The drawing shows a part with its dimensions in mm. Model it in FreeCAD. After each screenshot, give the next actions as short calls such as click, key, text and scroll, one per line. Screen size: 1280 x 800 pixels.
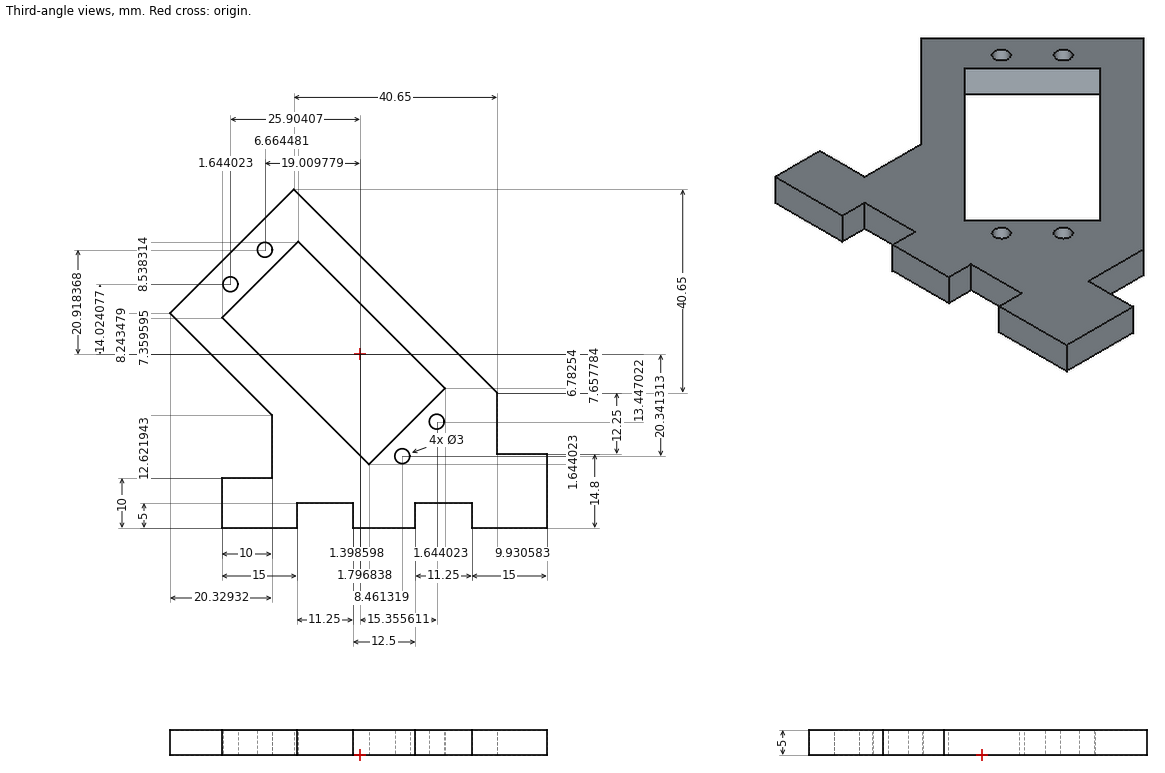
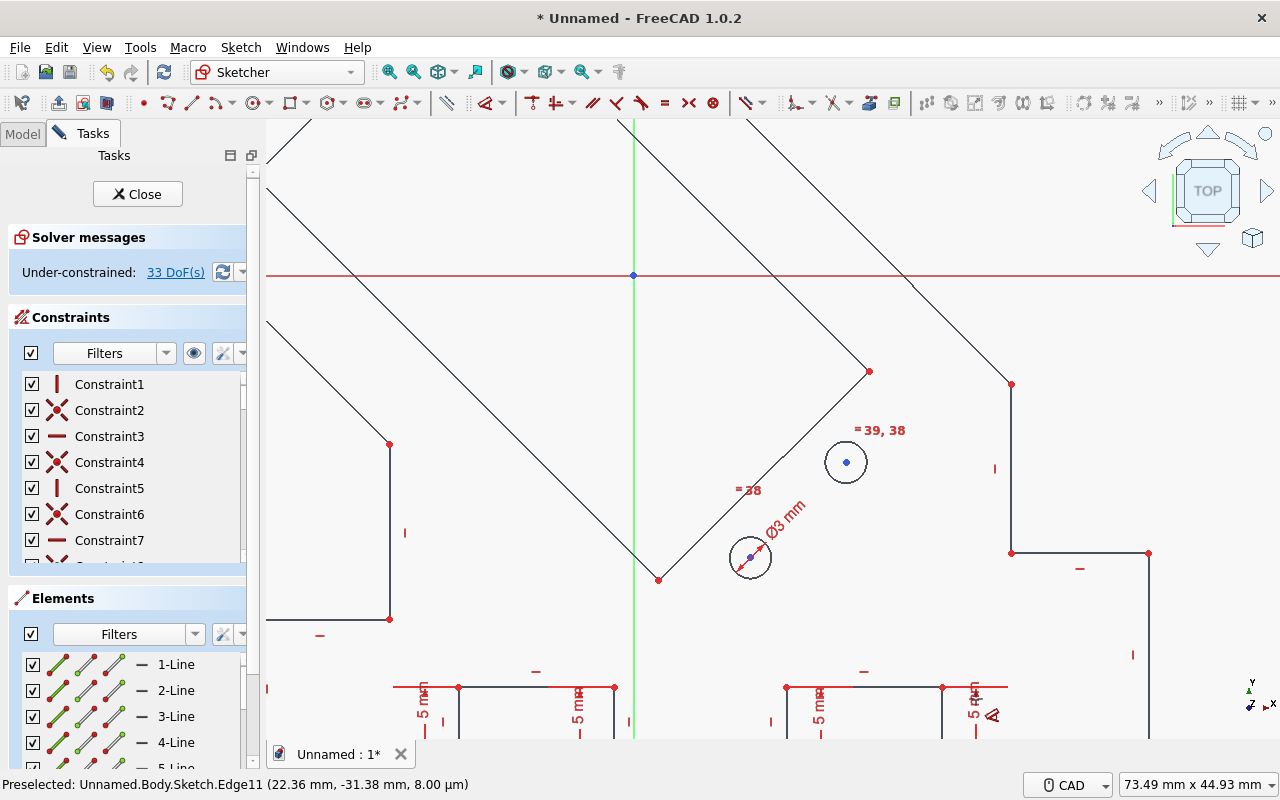
click(348, 620)
click(342, 654)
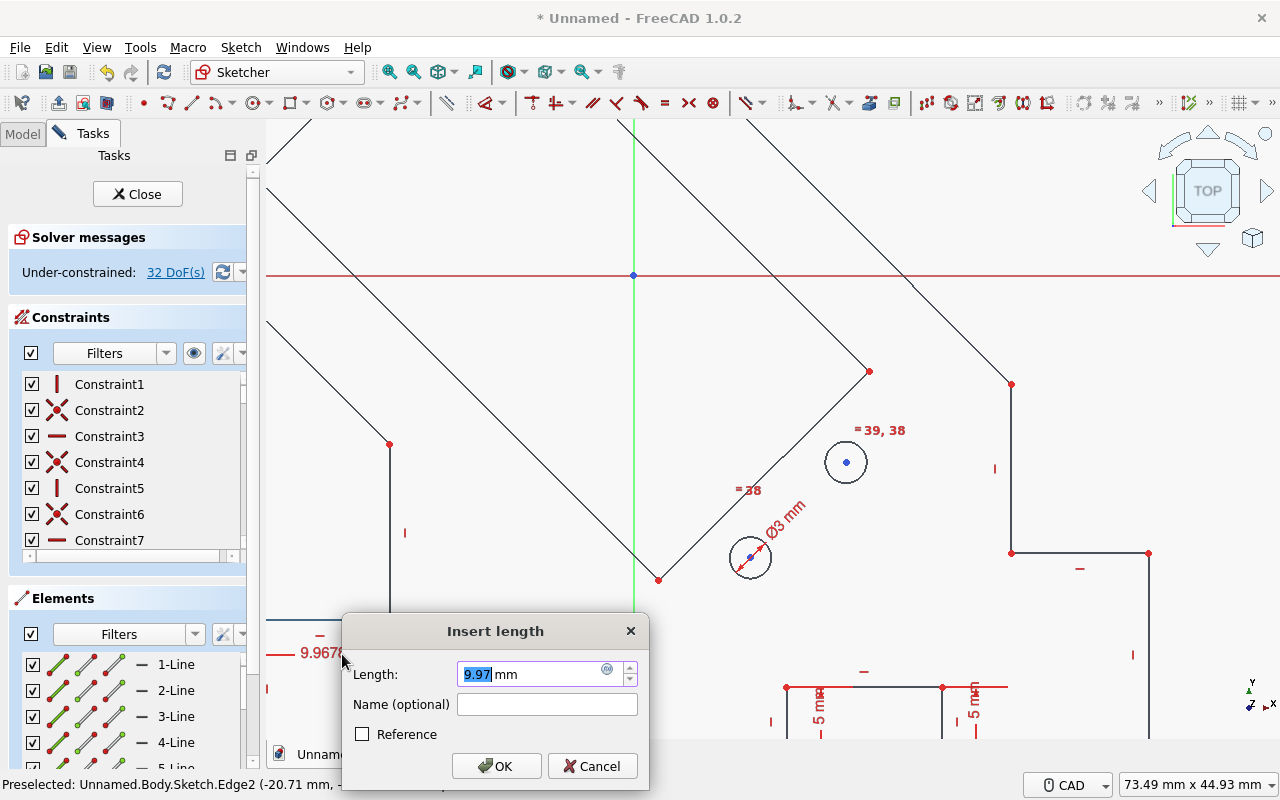
text(10)
key(Return)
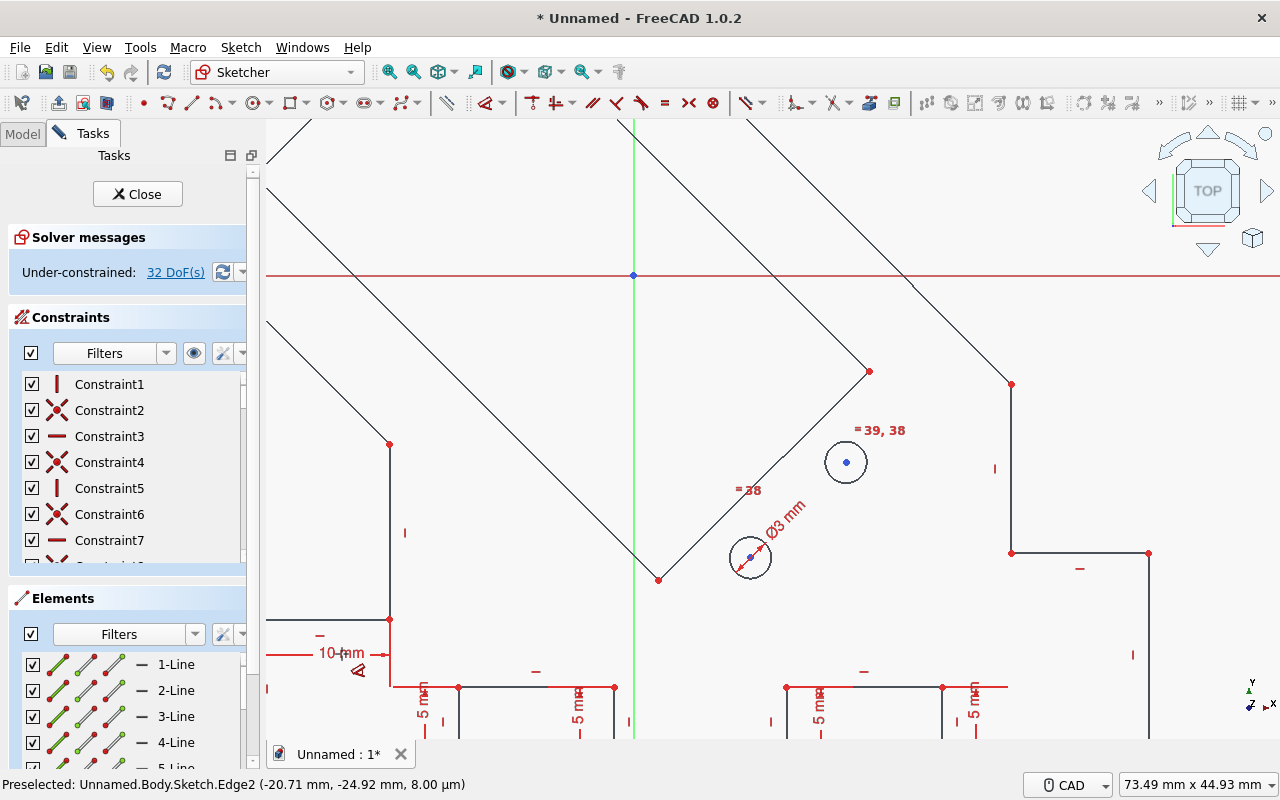
scroll(766, 544, down, 4)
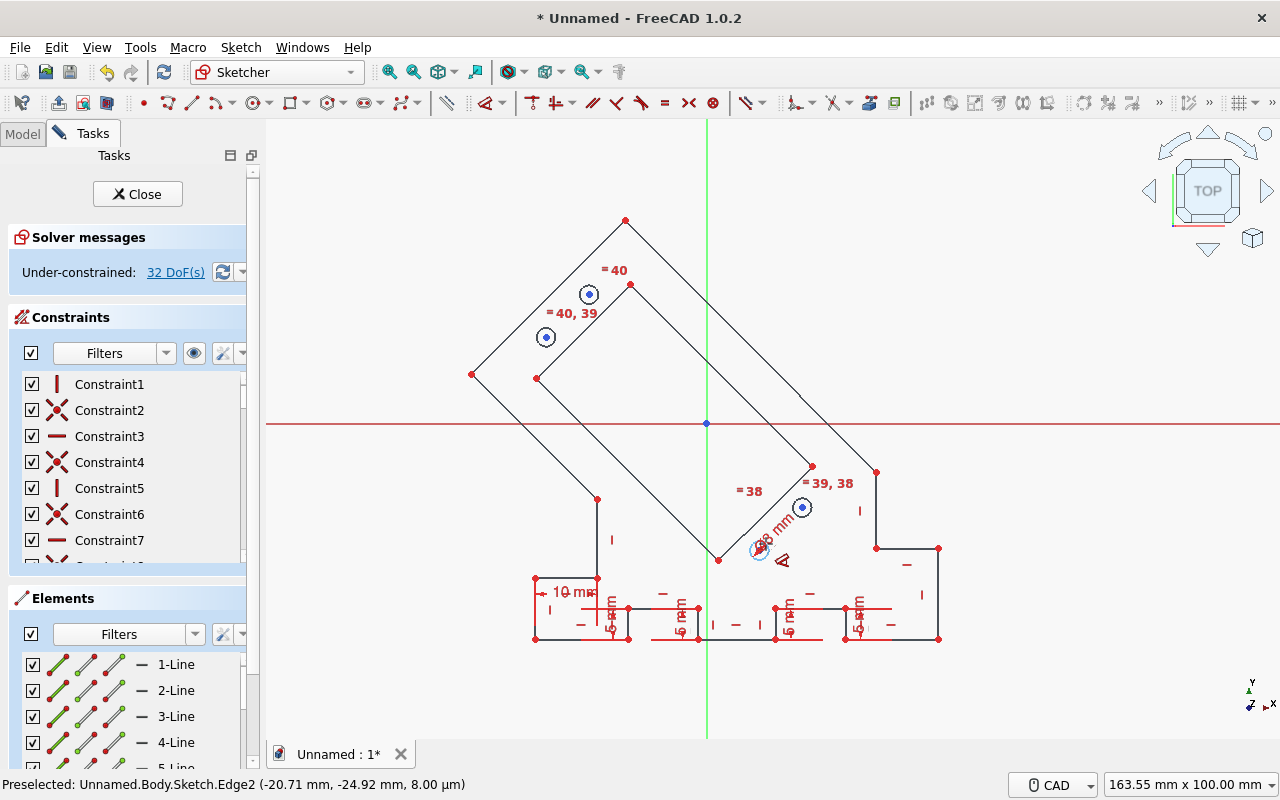
click(535, 597)
click(501, 609)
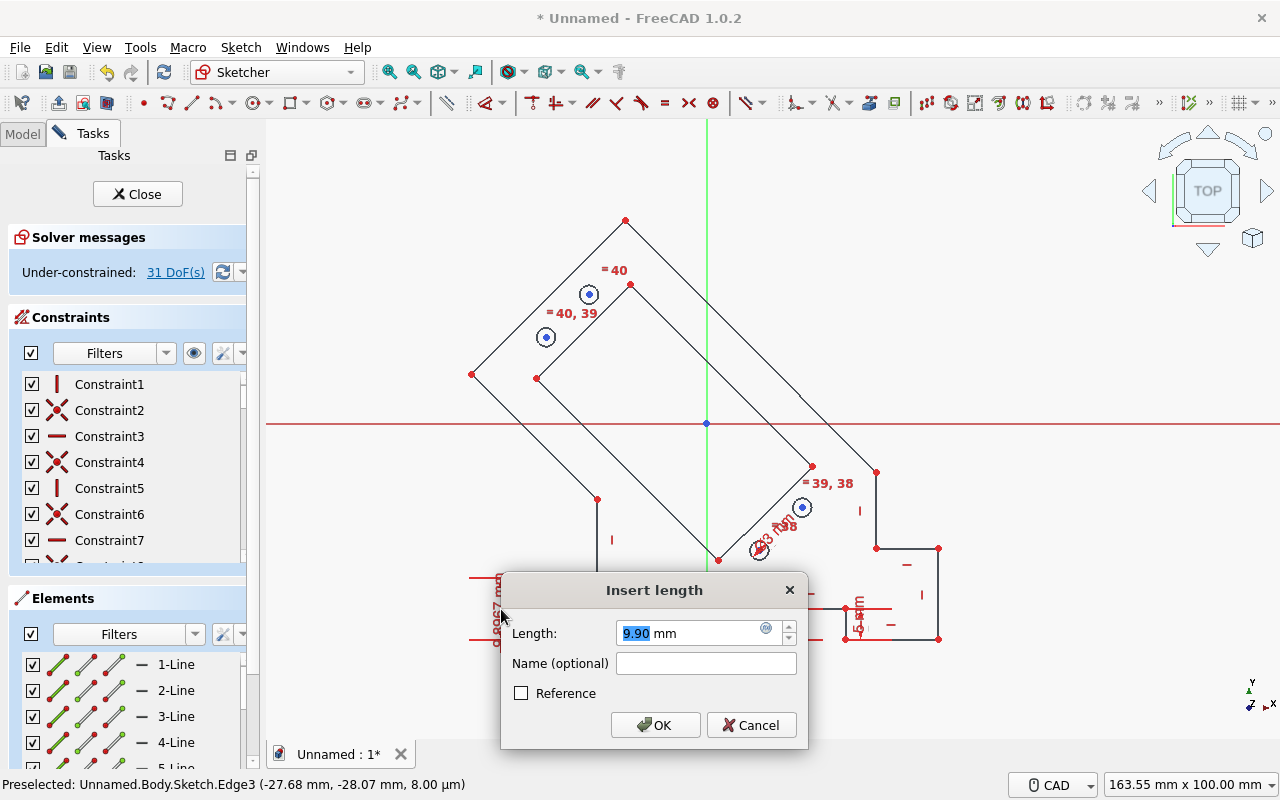
text(10)
key(Return)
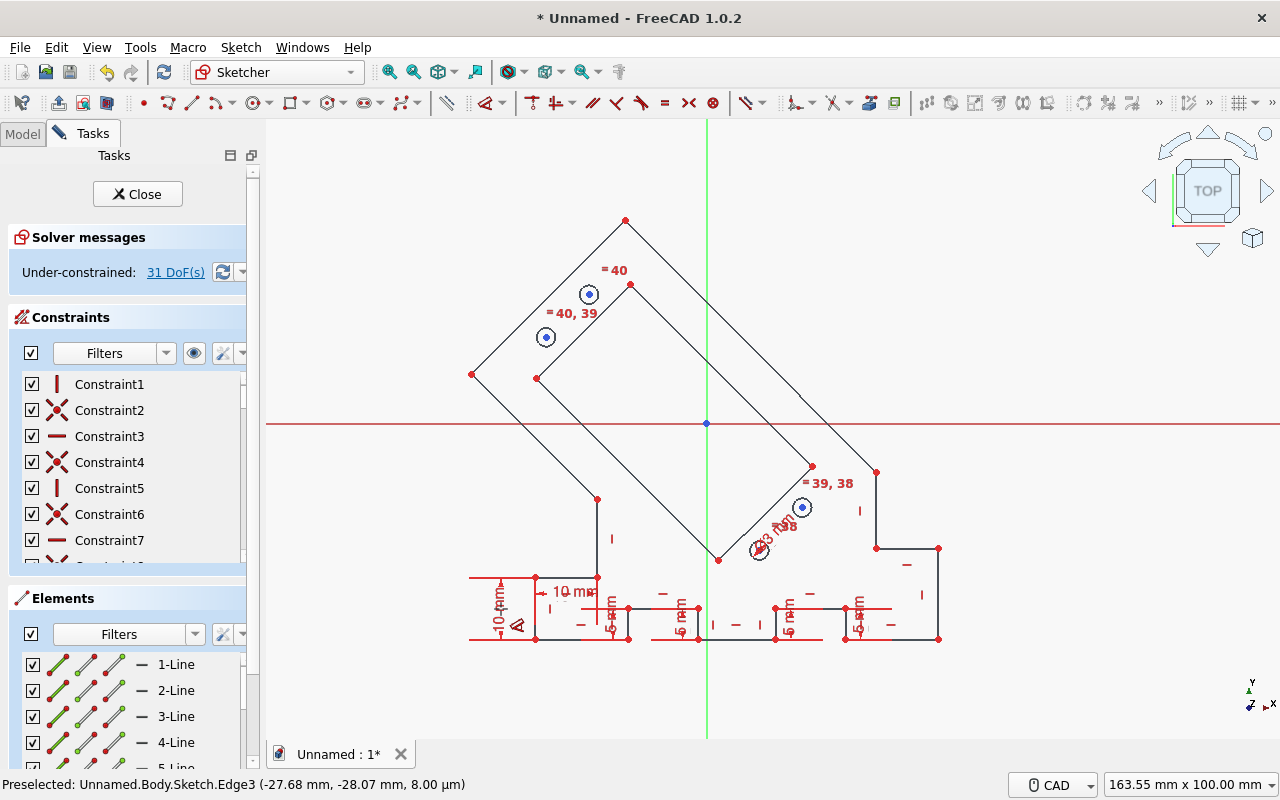
click(563, 640)
click(582, 674)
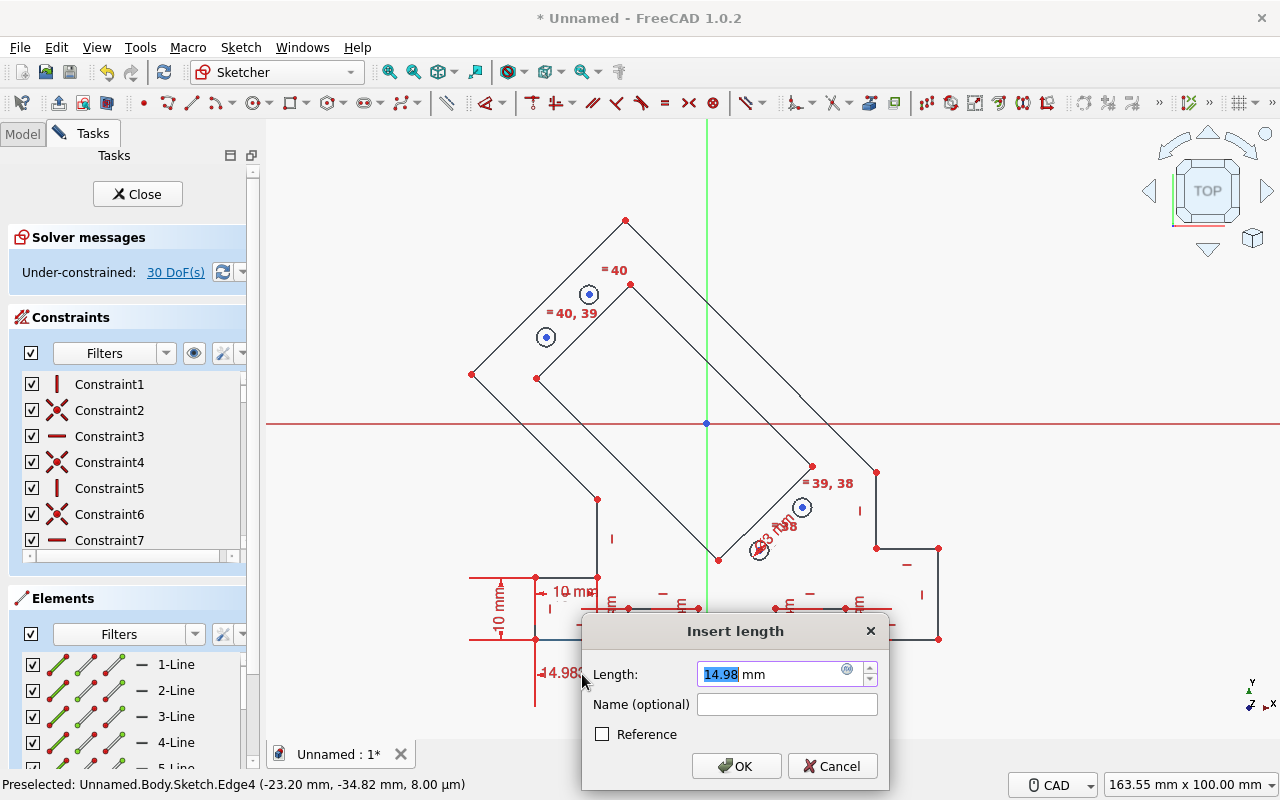
text(15)
key(Return)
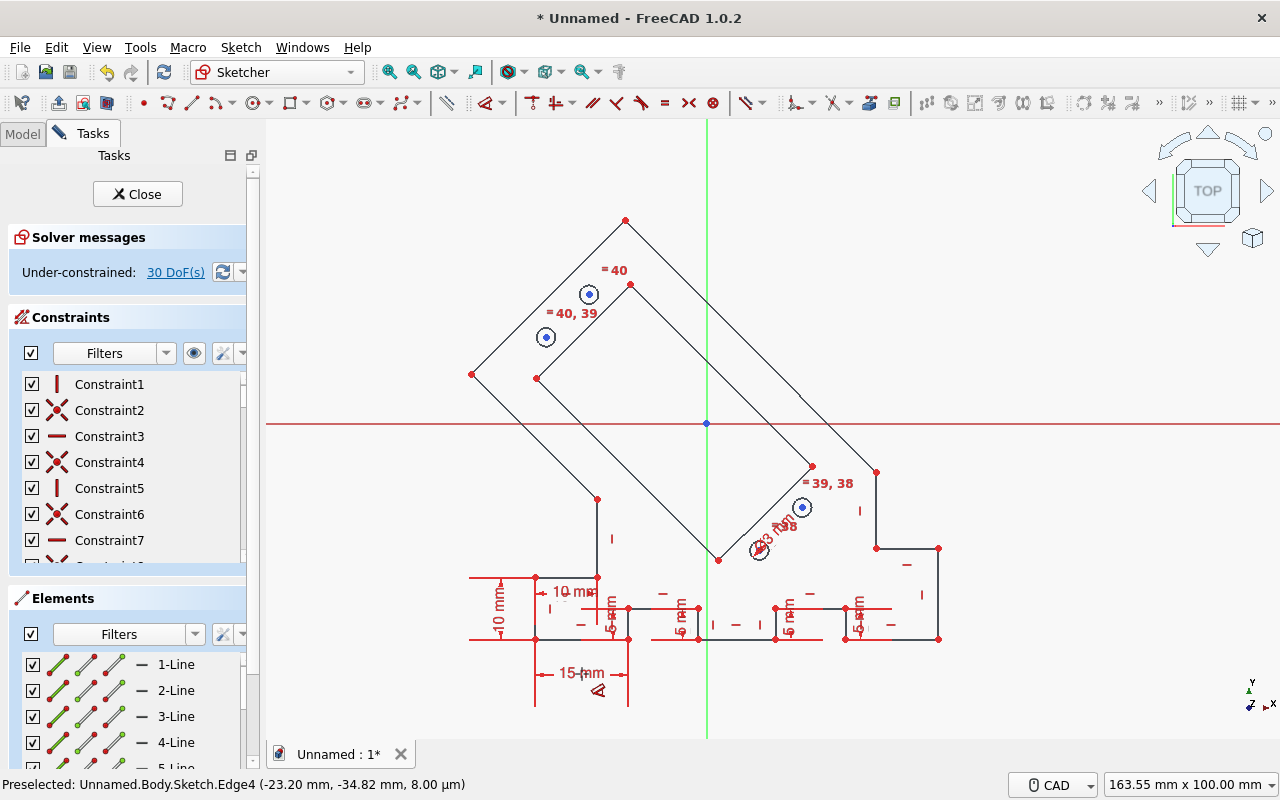
click(873, 640)
click(892, 674)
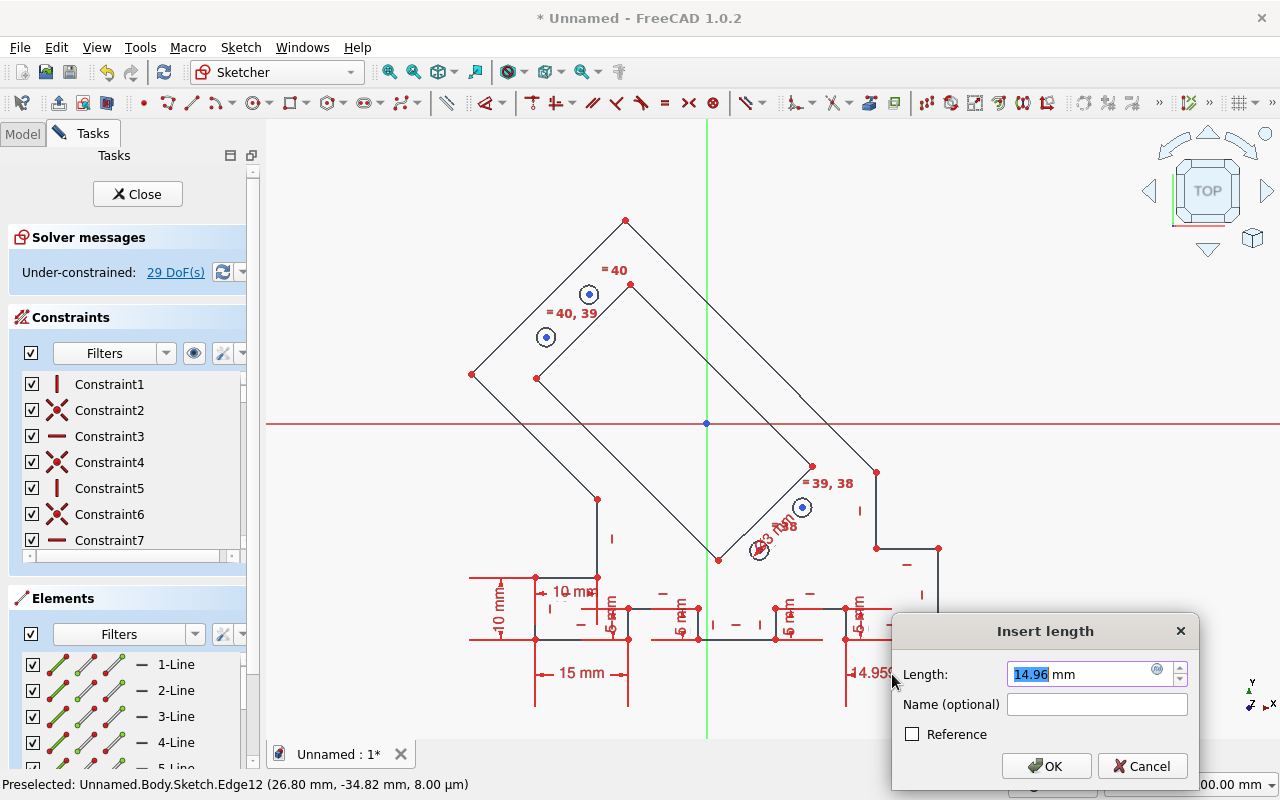
text(15)
key(Return)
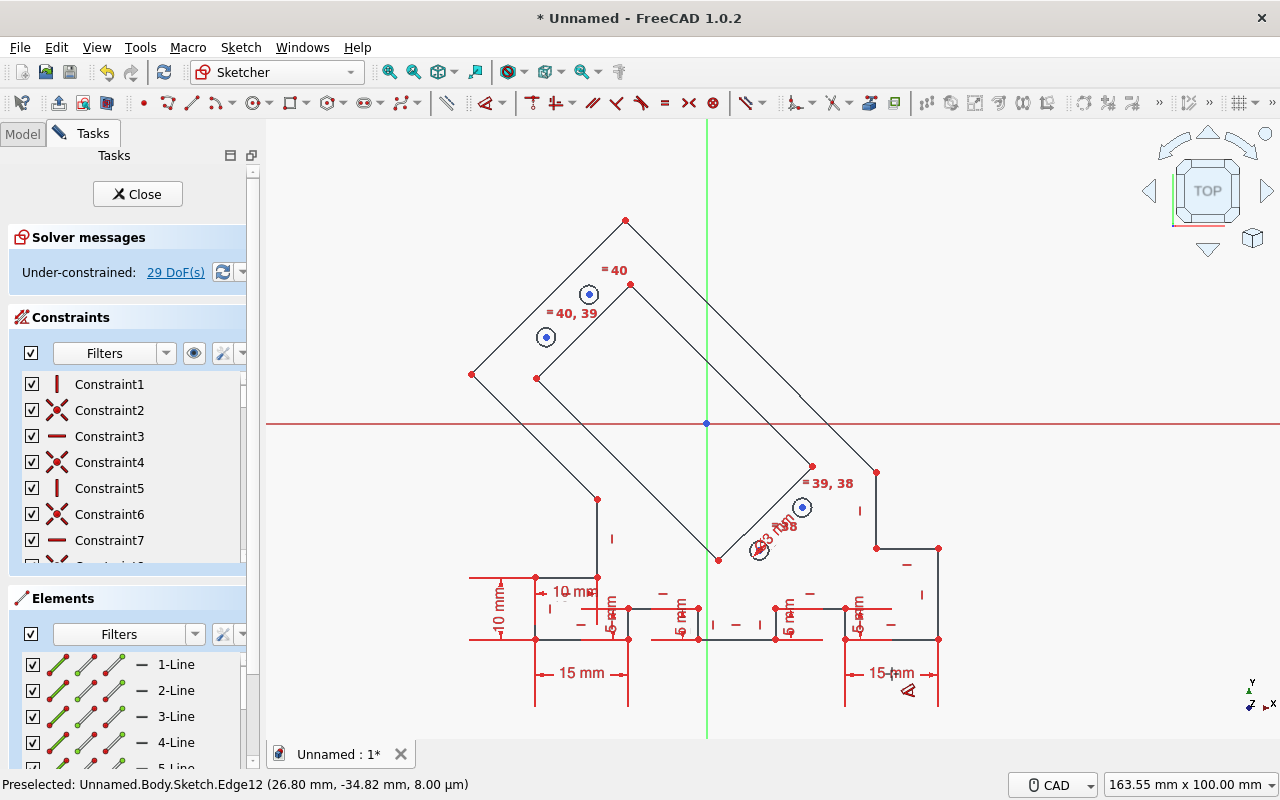
click(721, 640)
click(737, 674)